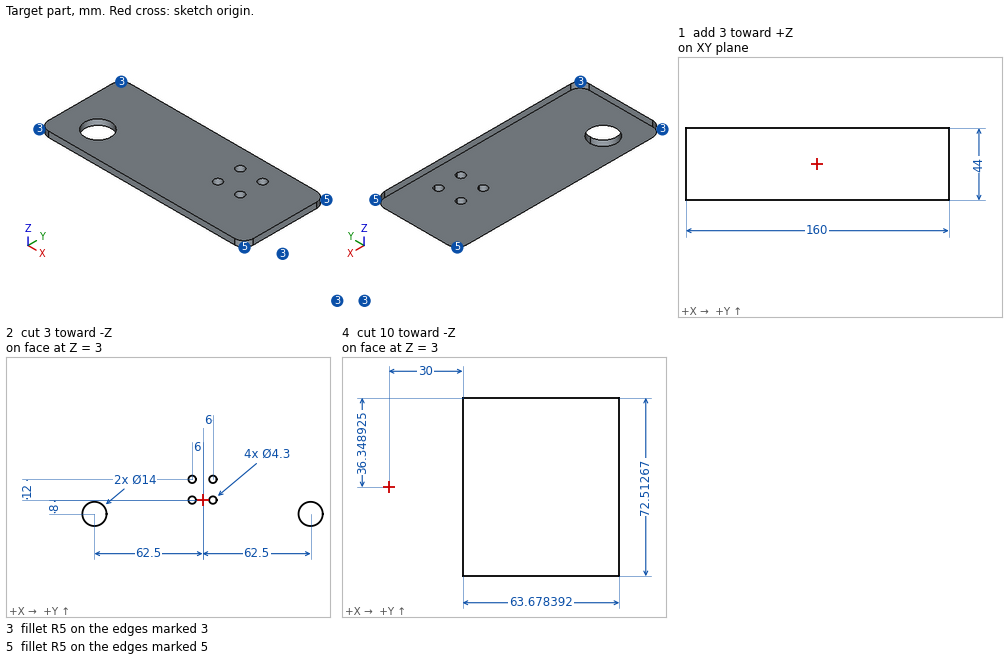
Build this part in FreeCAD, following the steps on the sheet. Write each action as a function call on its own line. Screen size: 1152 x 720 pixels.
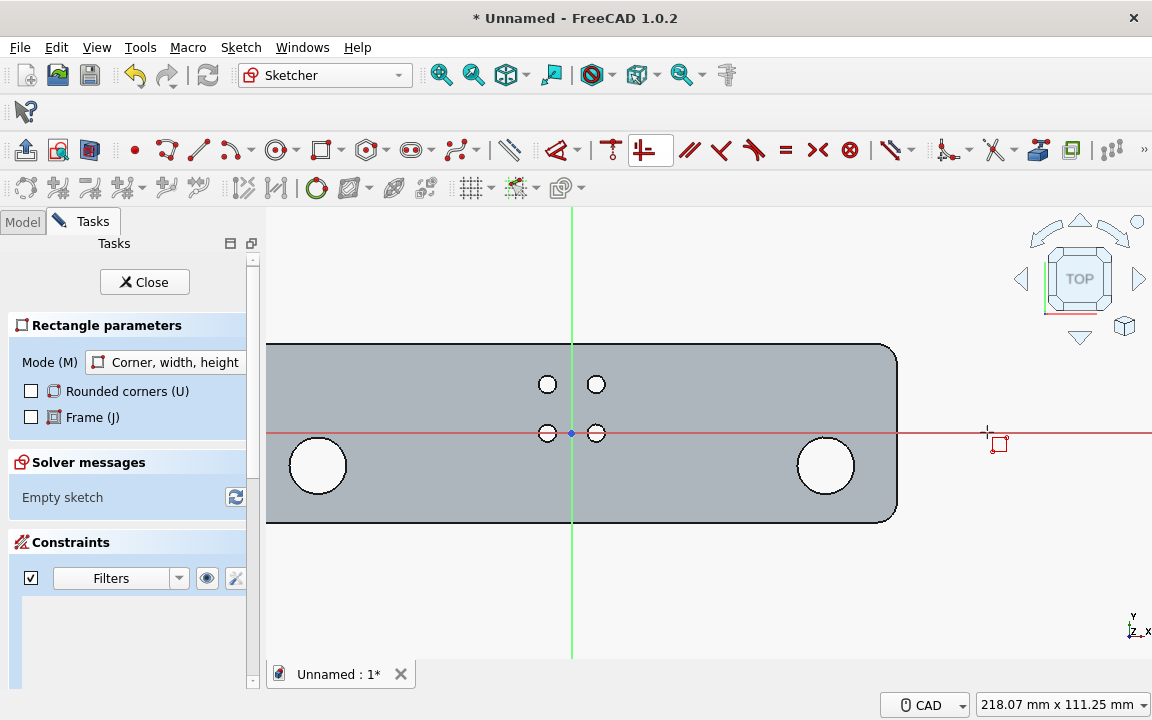
click(694, 286)
move(952, 580)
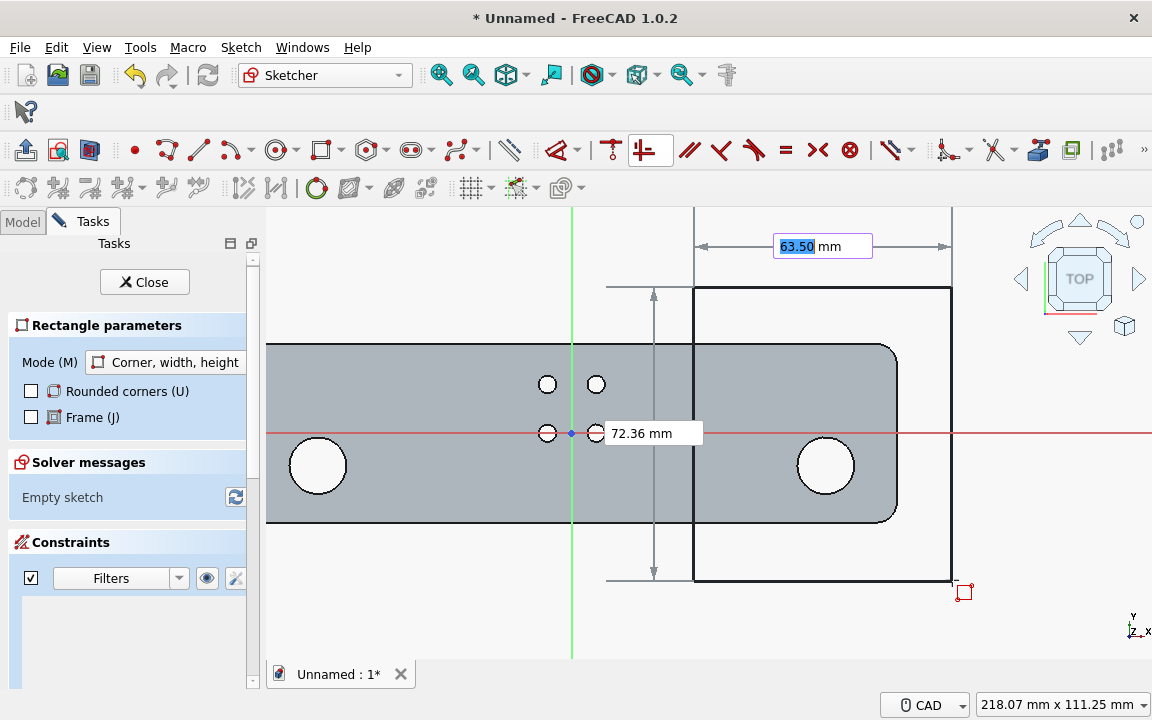
text(63.678392)
key(Tab)
text(72.51267)
key(Return)
key(Escape)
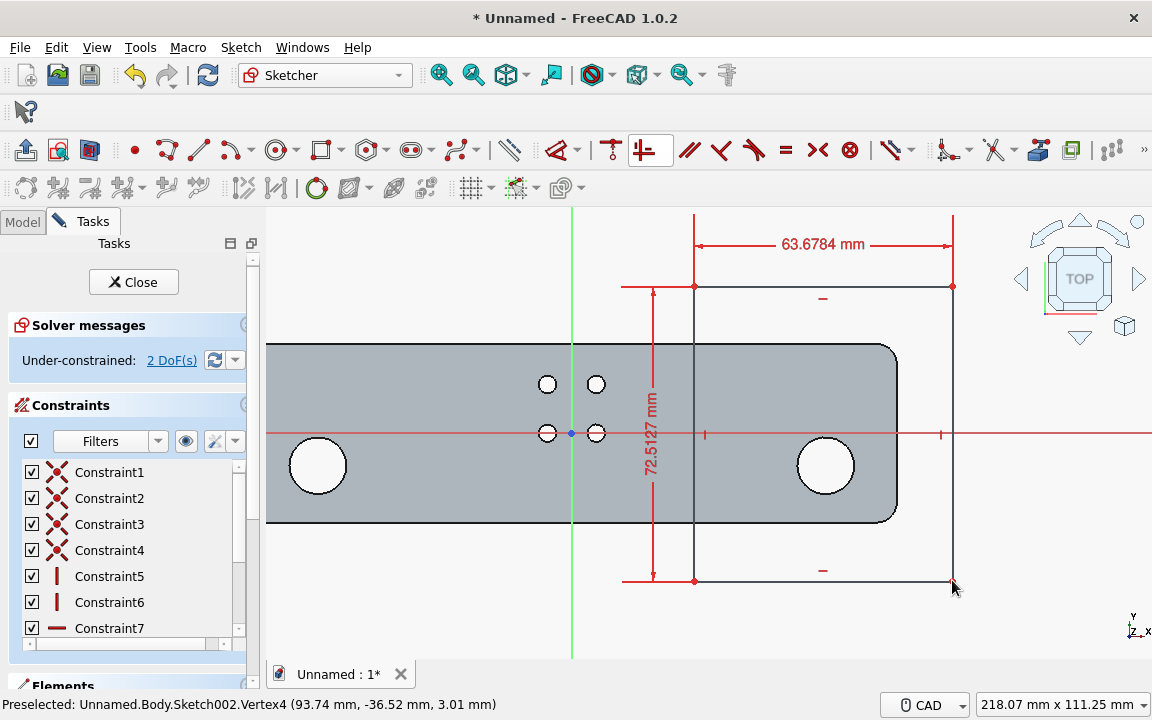
key(d)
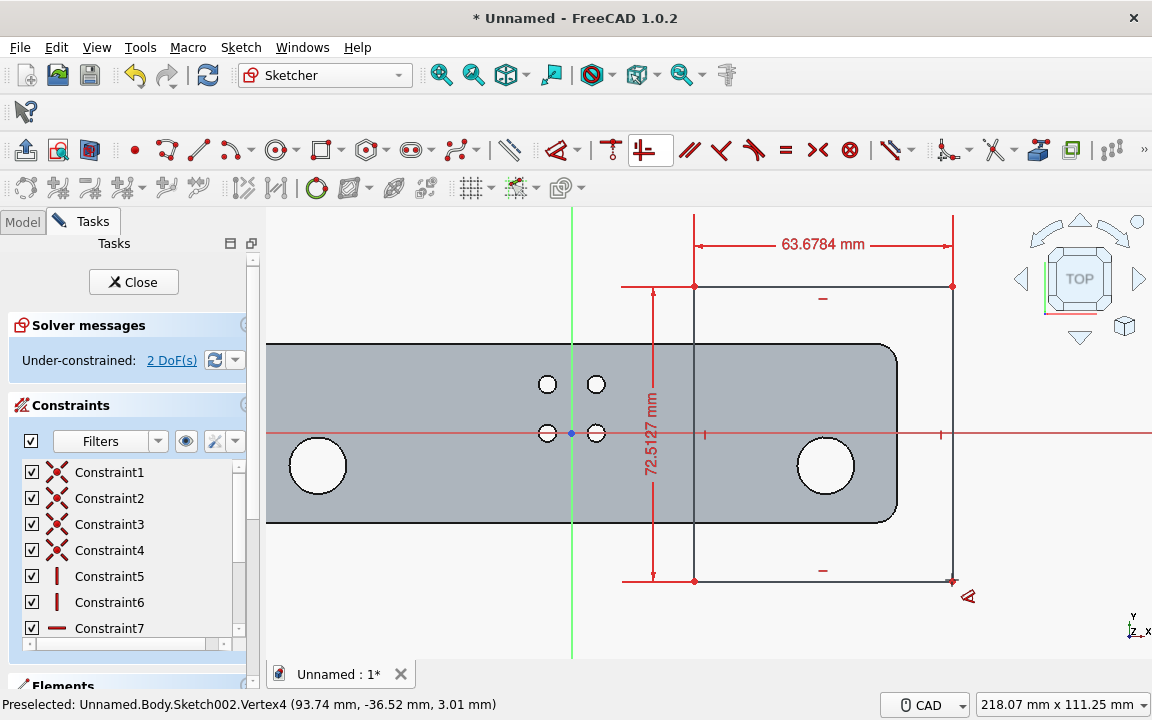
click(694, 287)
click(633, 253)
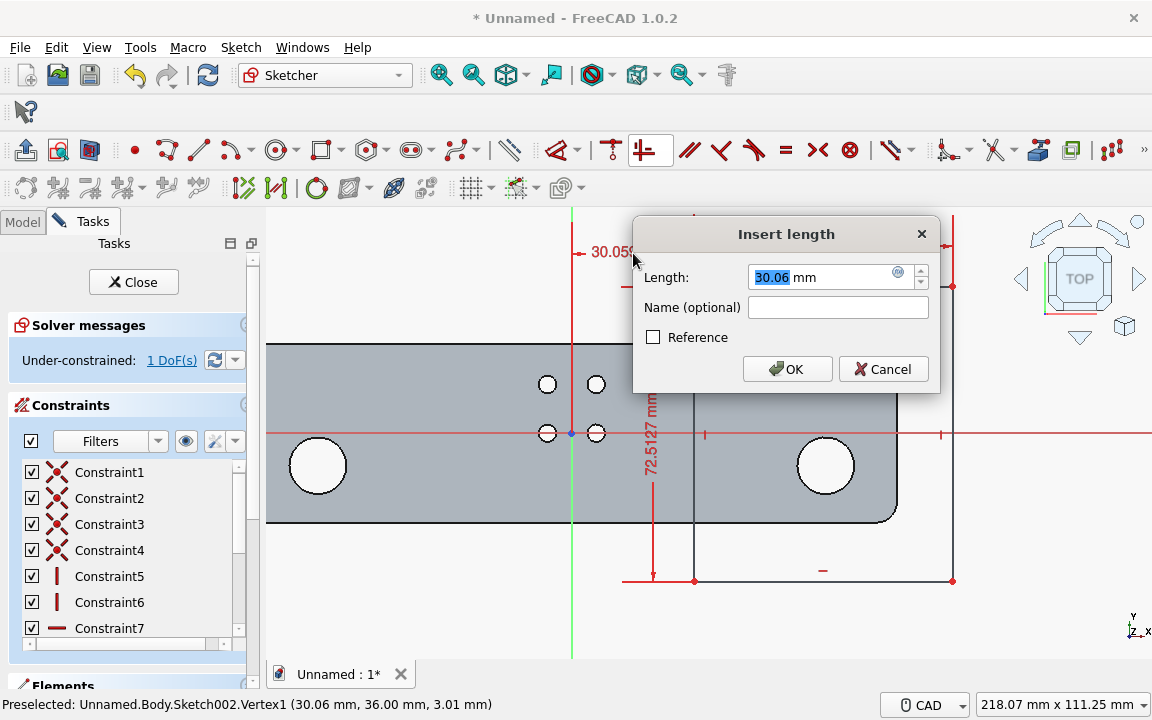
text(30)
key(Return)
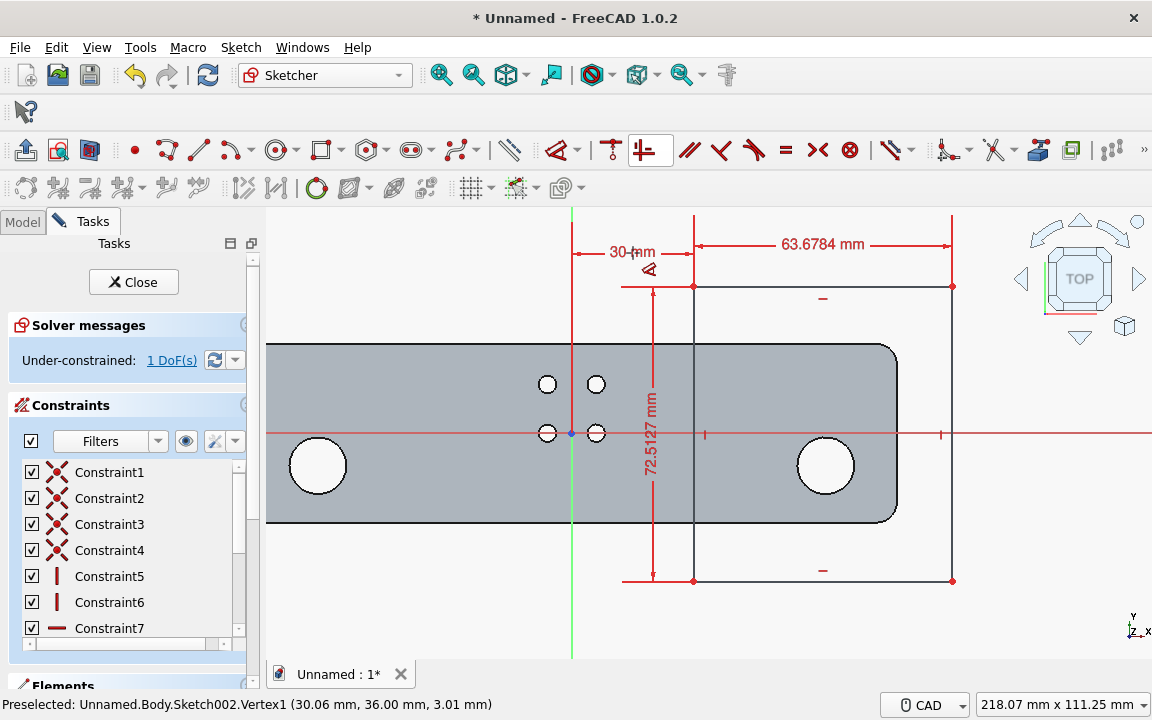
click(694, 287)
click(538, 360)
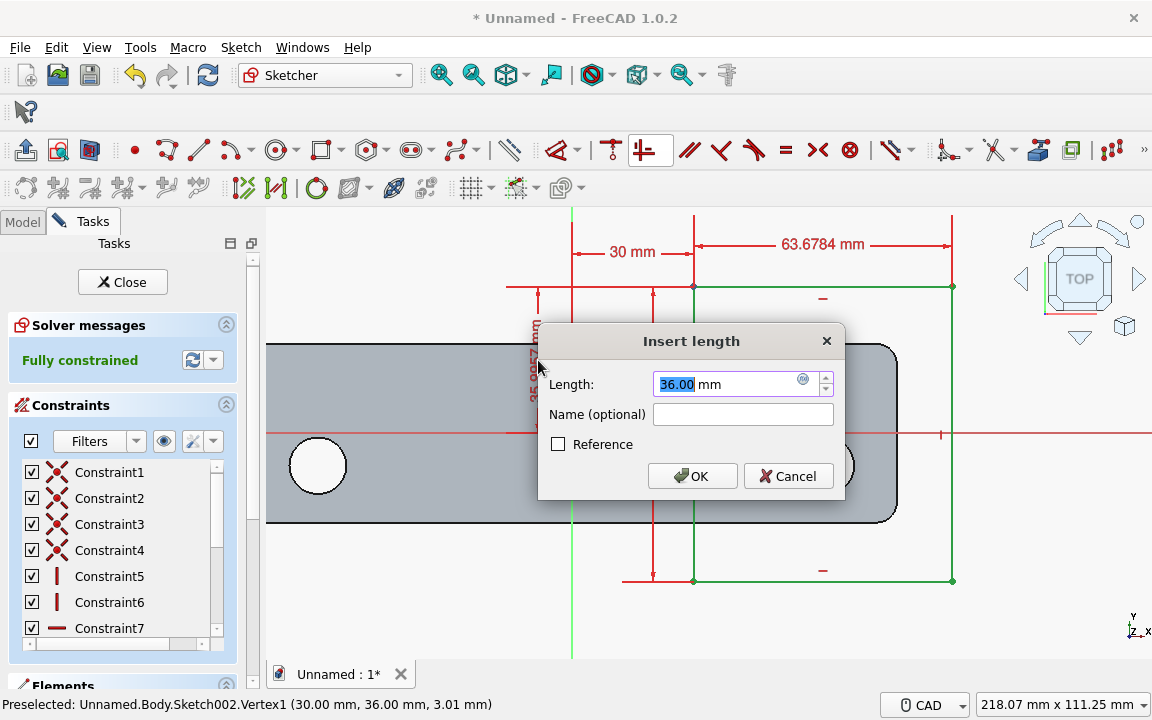
text(36.348925)
key(Return)
key(Escape)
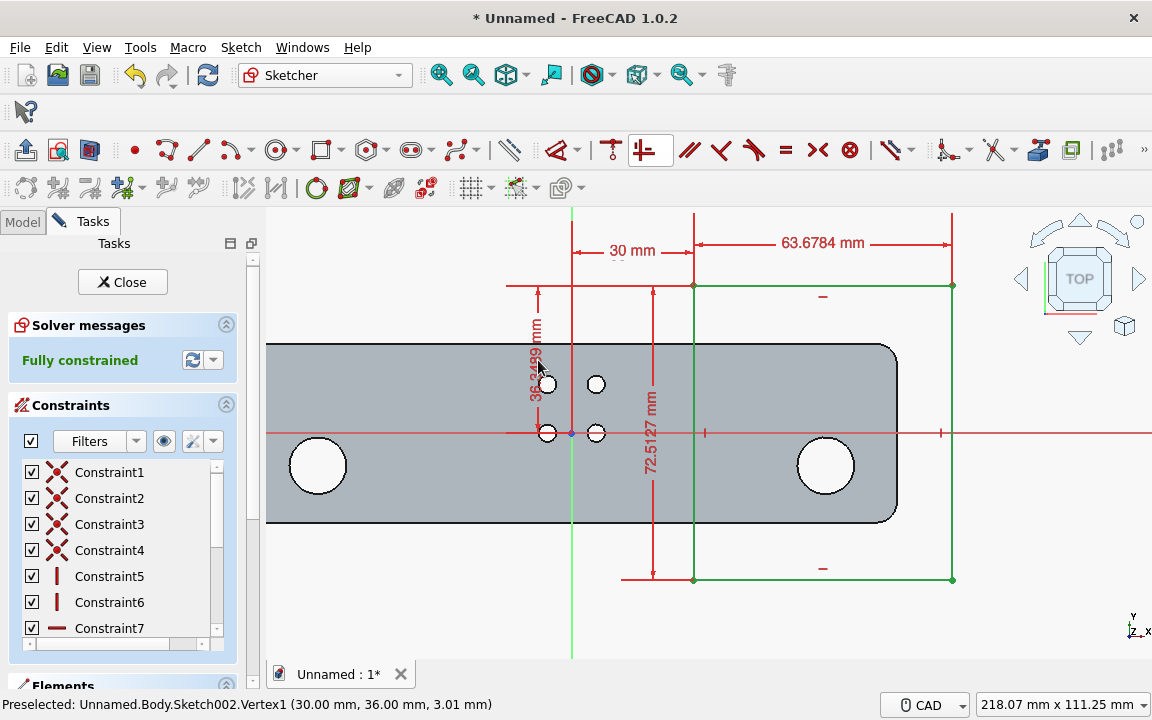
click(123, 282)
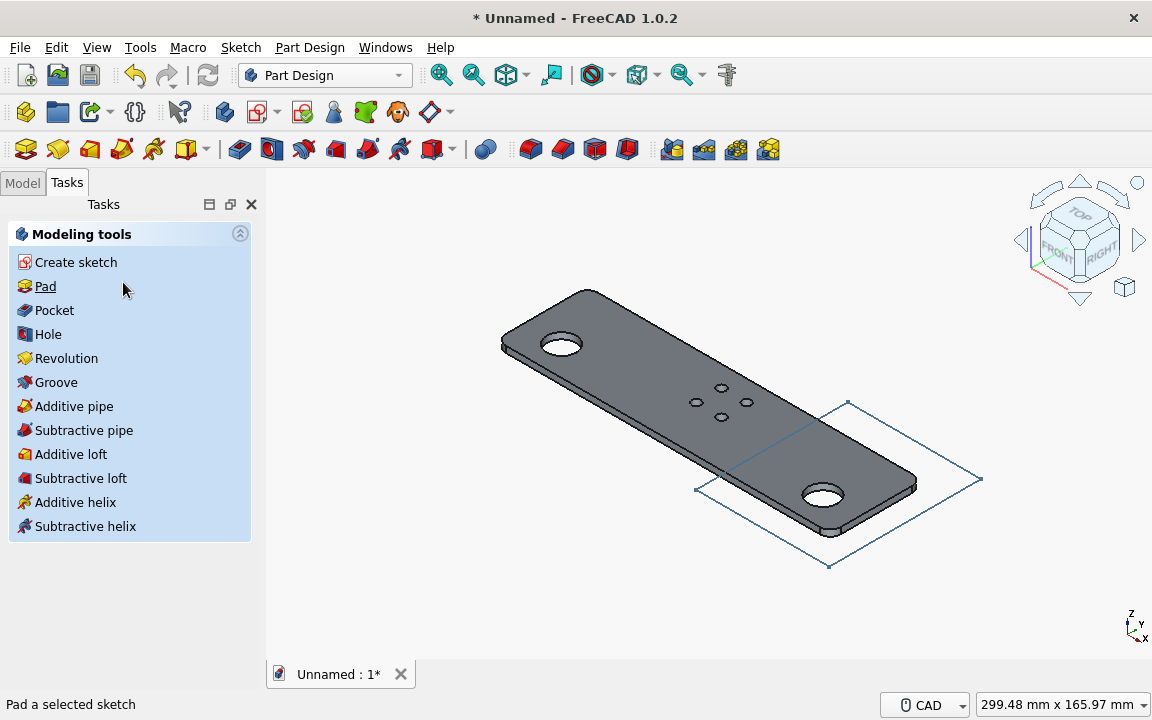
click(240, 150)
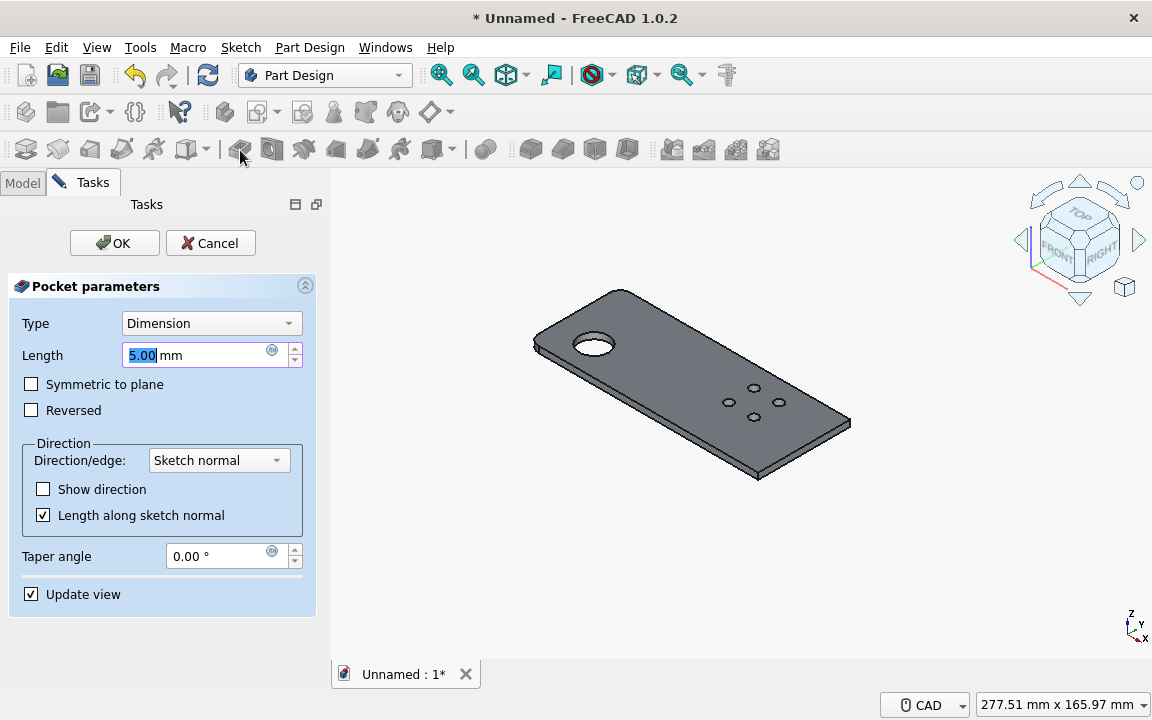
text(10)
key(Tab)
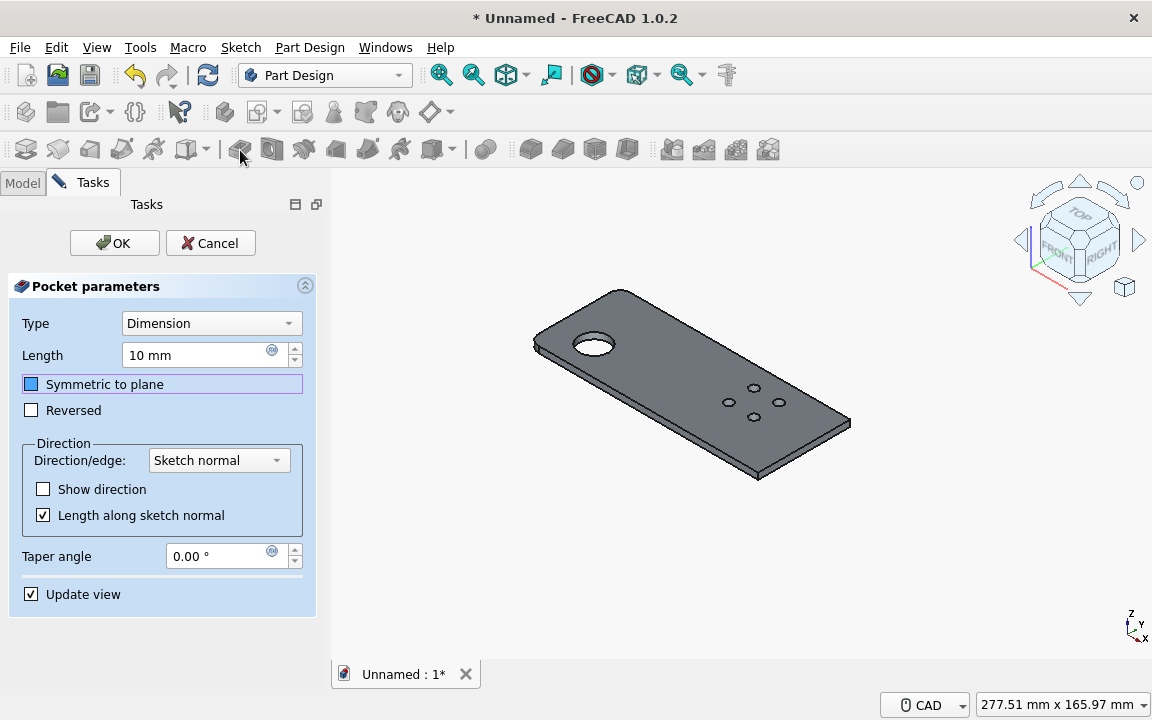
click(115, 243)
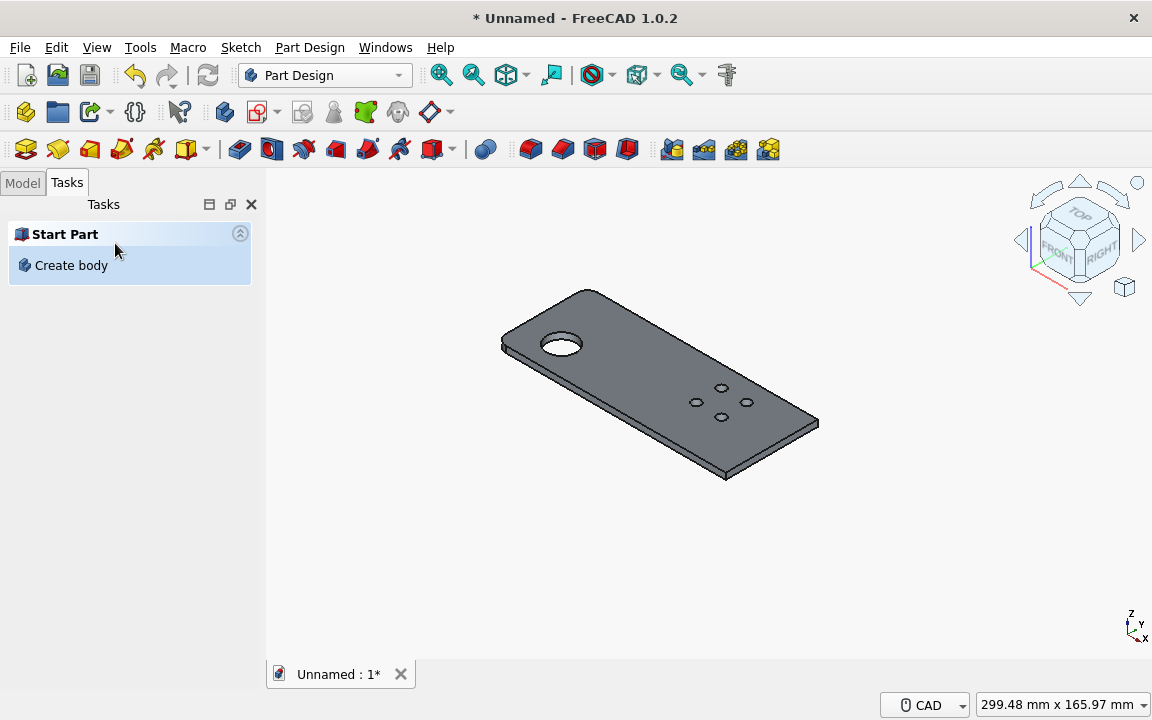
key(v)
key(f)